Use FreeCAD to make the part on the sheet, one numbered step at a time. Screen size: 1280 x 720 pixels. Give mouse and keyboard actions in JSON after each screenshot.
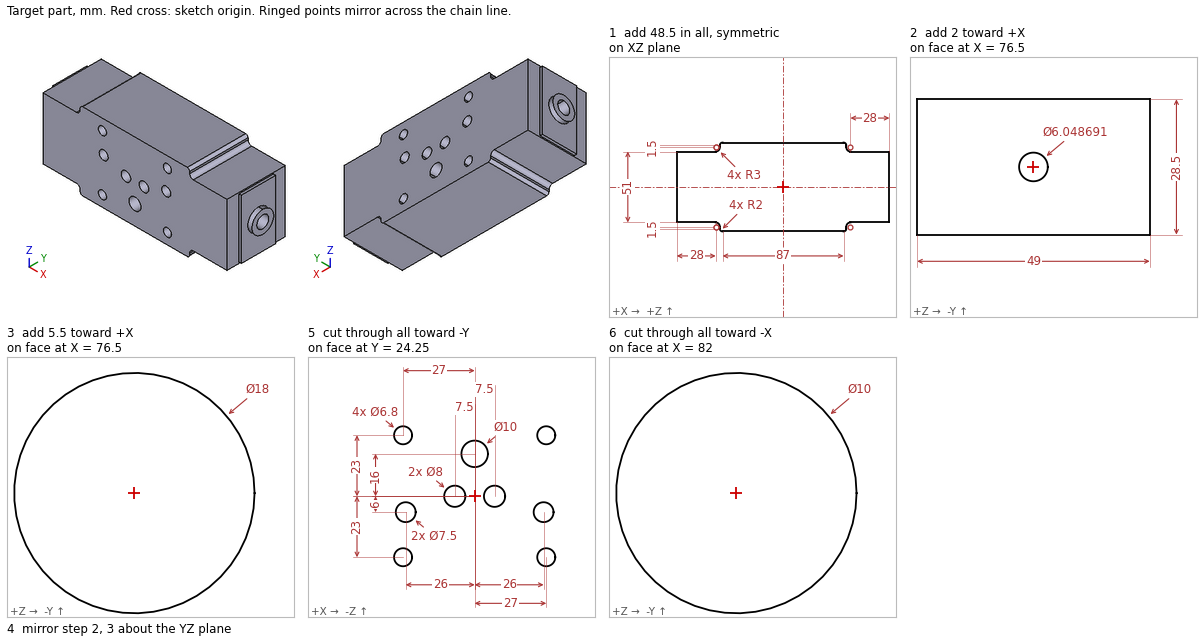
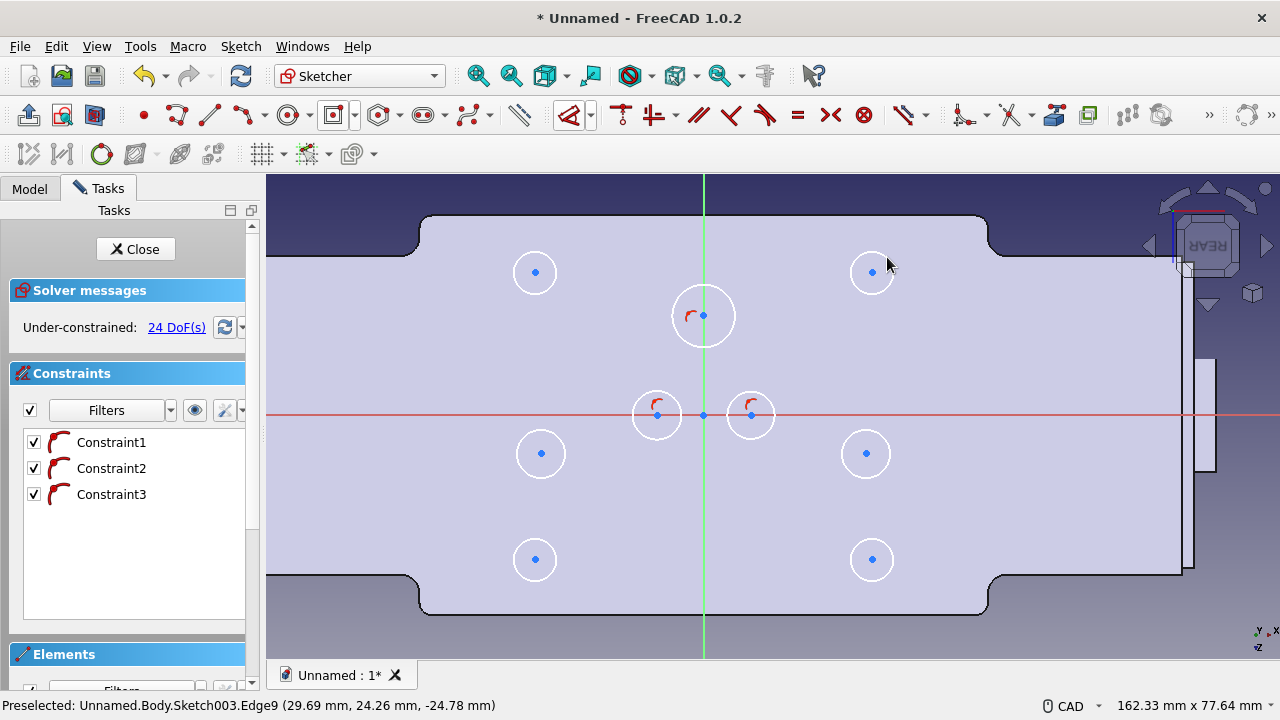
{"action": "left_click", "coordinate": [550, 258]}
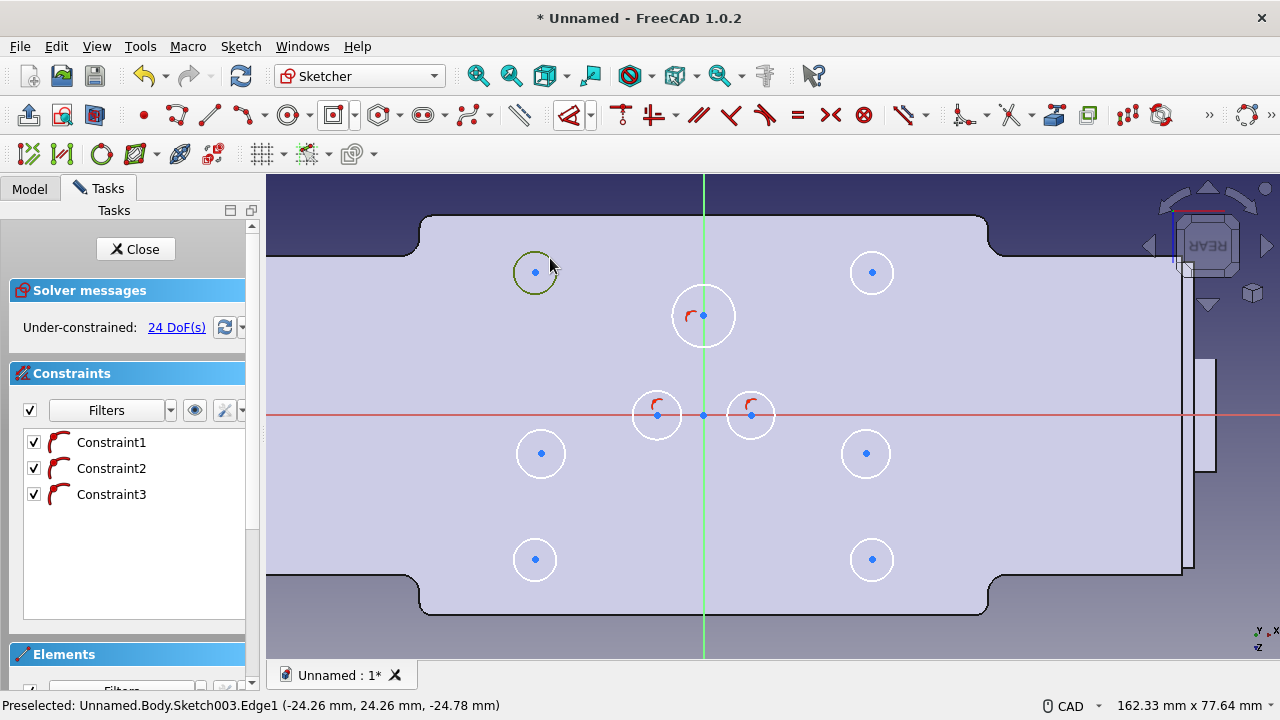
{"action": "left_click", "coordinate": [550, 545]}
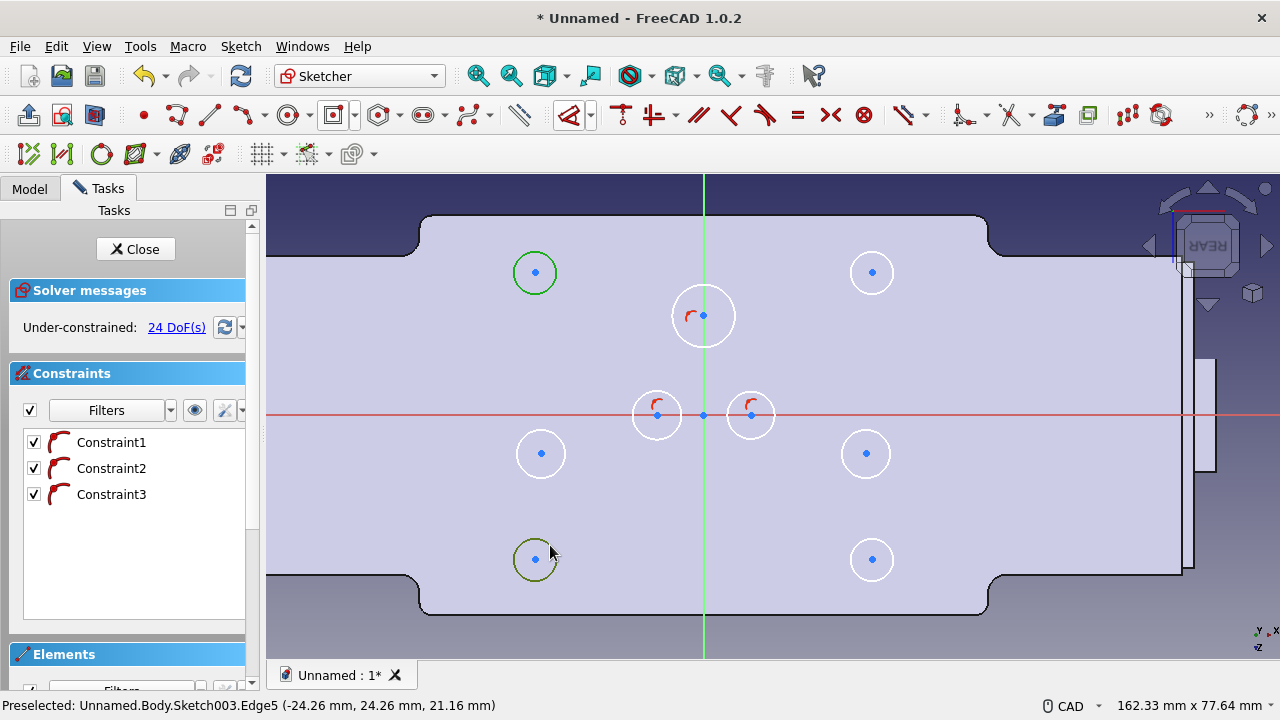
{"action": "left_click", "coordinate": [887, 545]}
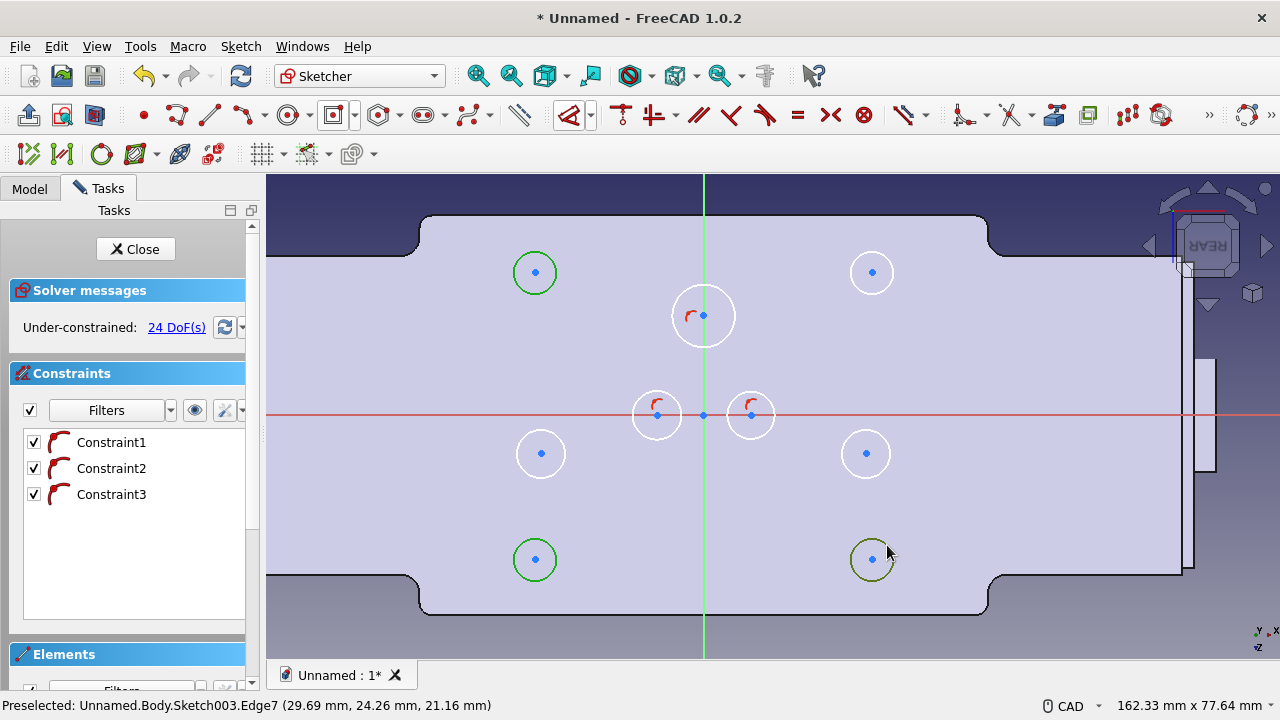
{"action": "left_click", "coordinate": [887, 258]}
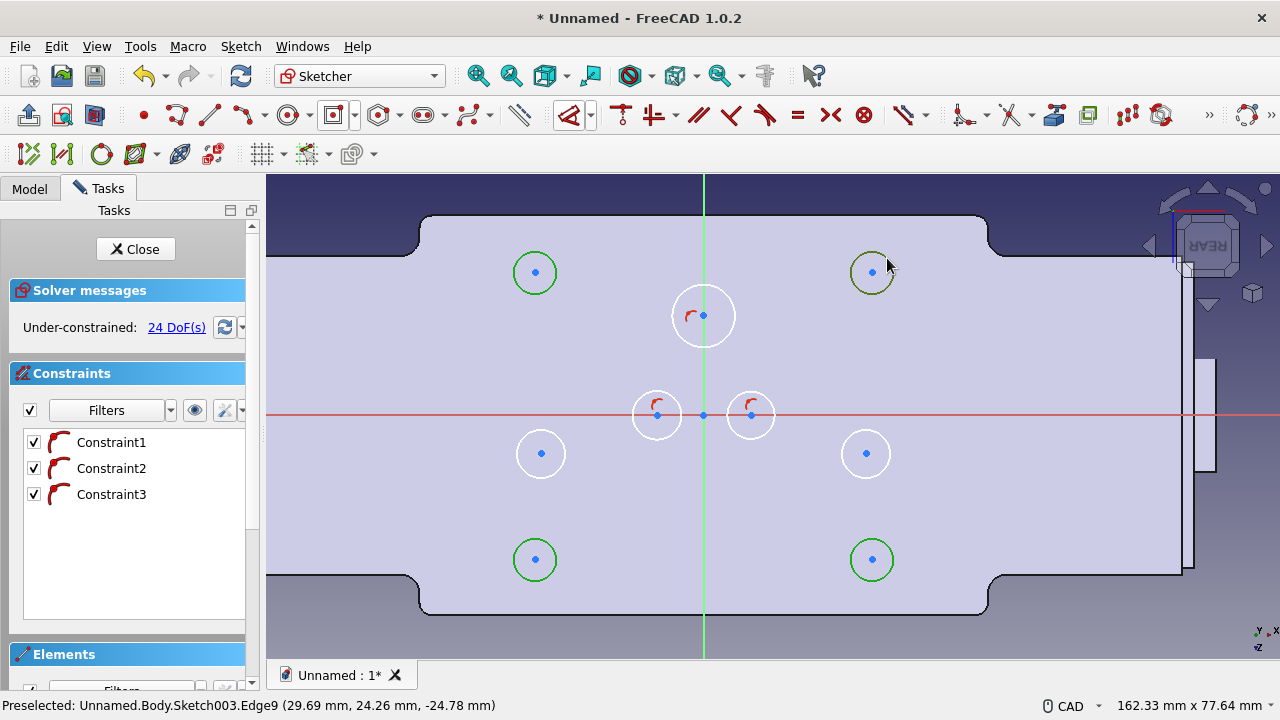
{"action": "left_click", "coordinate": [798, 116]}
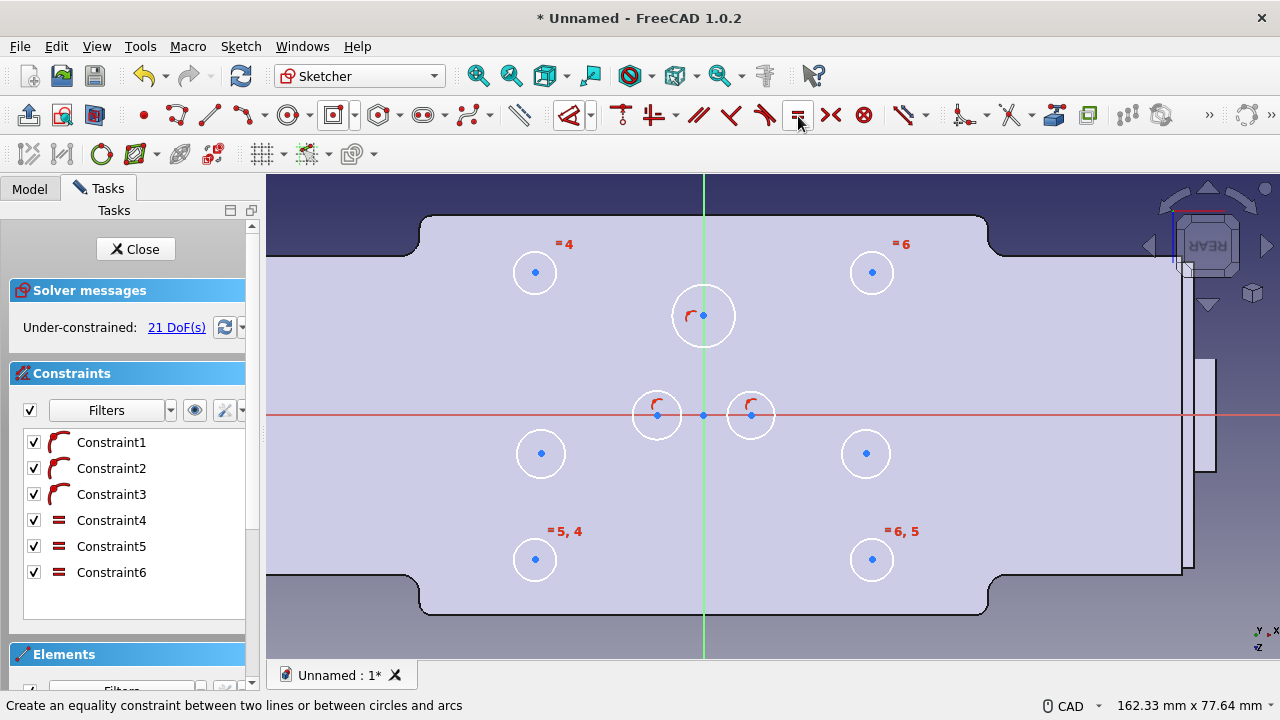
{"action": "left_click", "coordinate": [674, 398]}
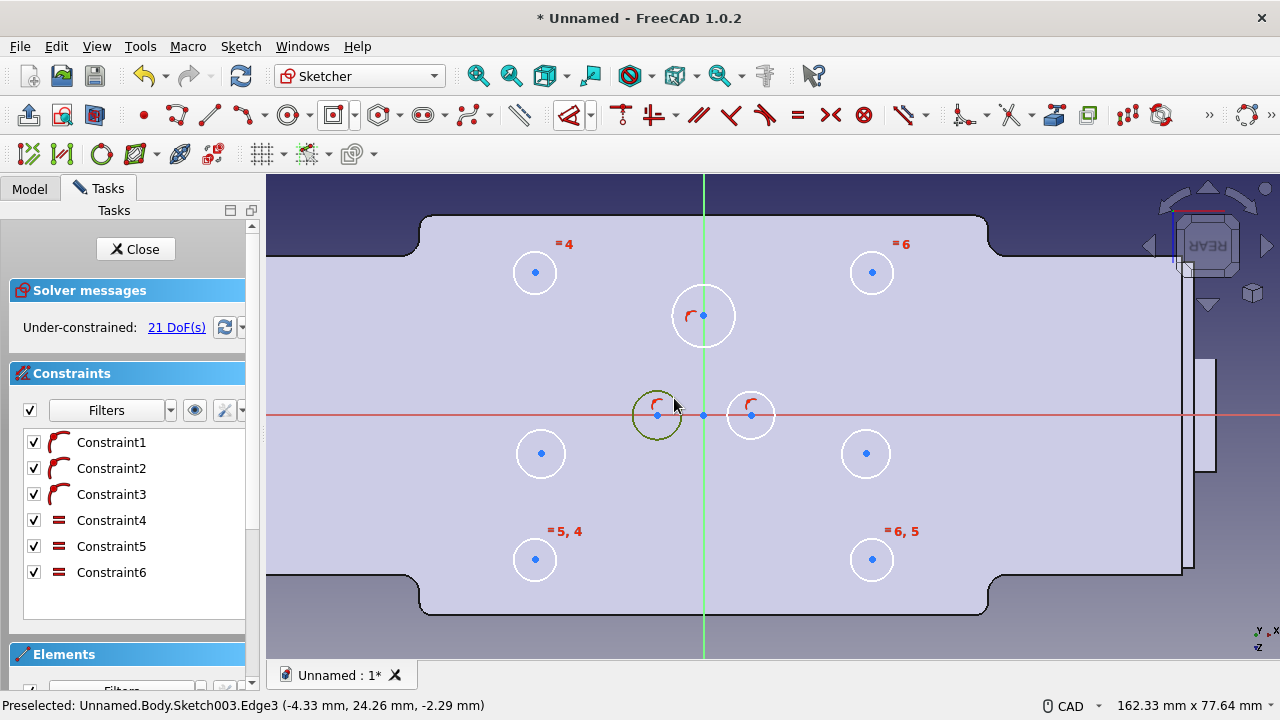
{"action": "left_click", "coordinate": [768, 399]}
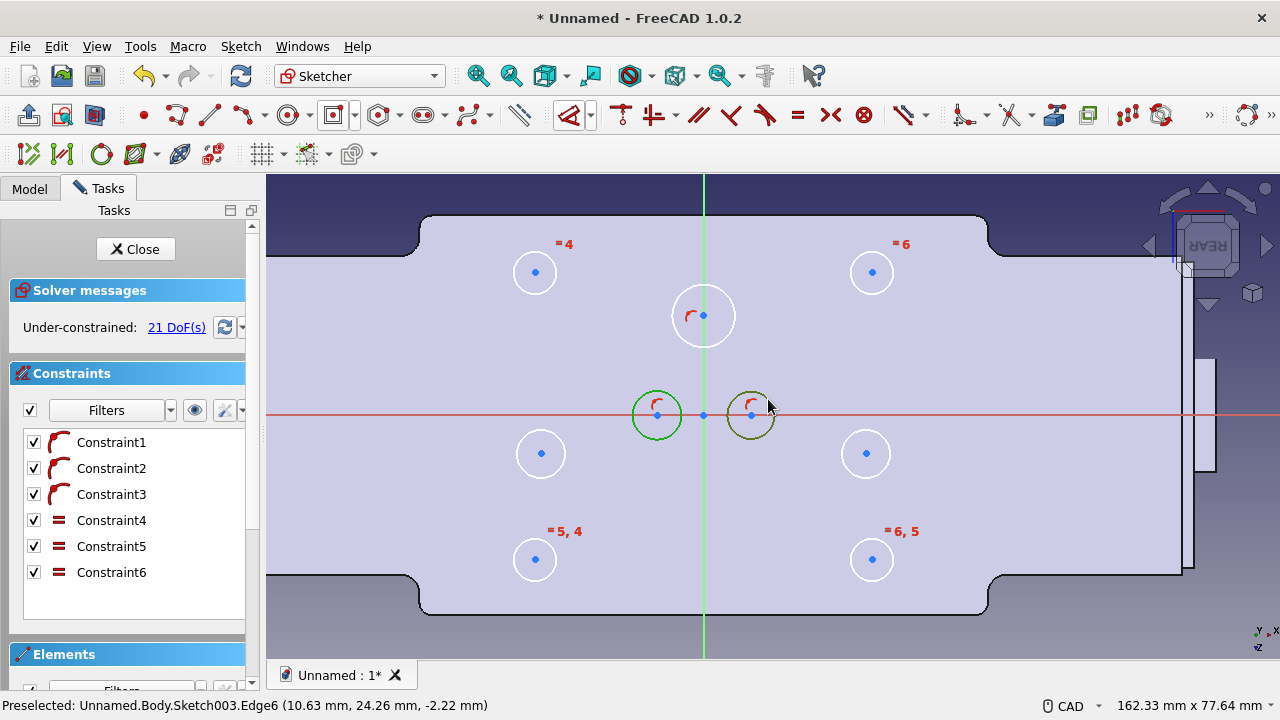
{"action": "left_click", "coordinate": [798, 116]}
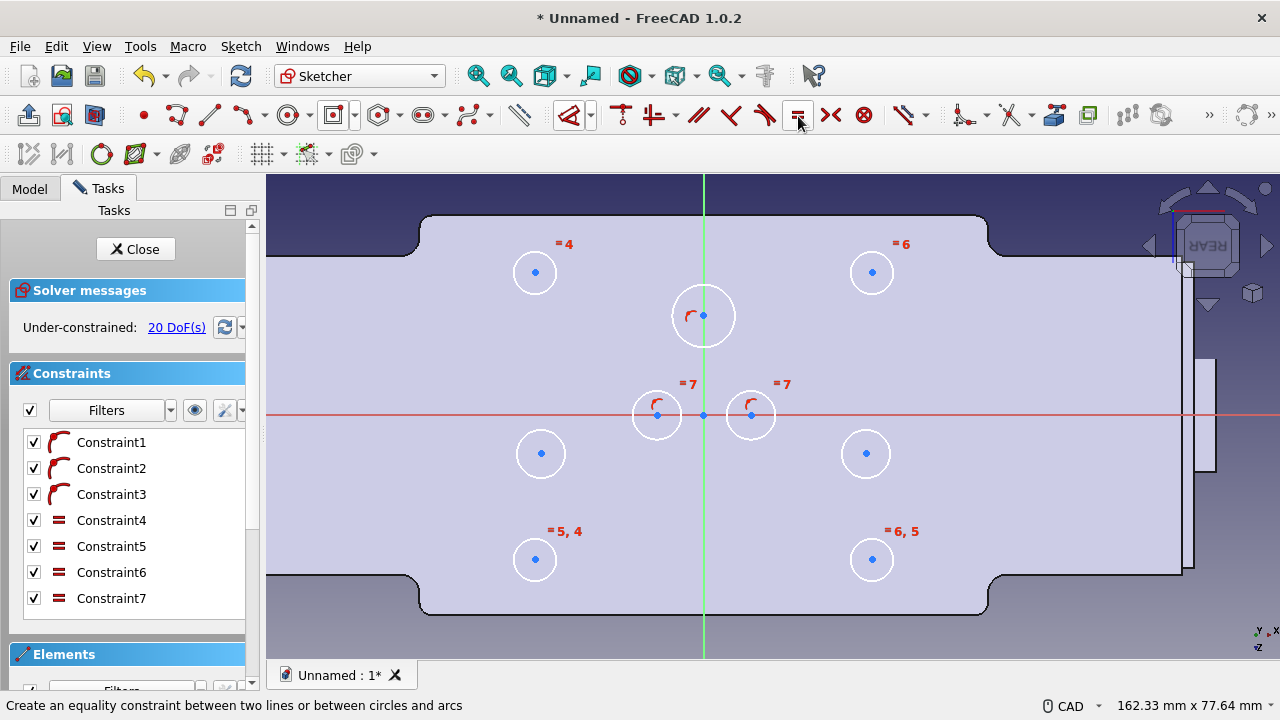
{"action": "left_click", "coordinate": [558, 437]}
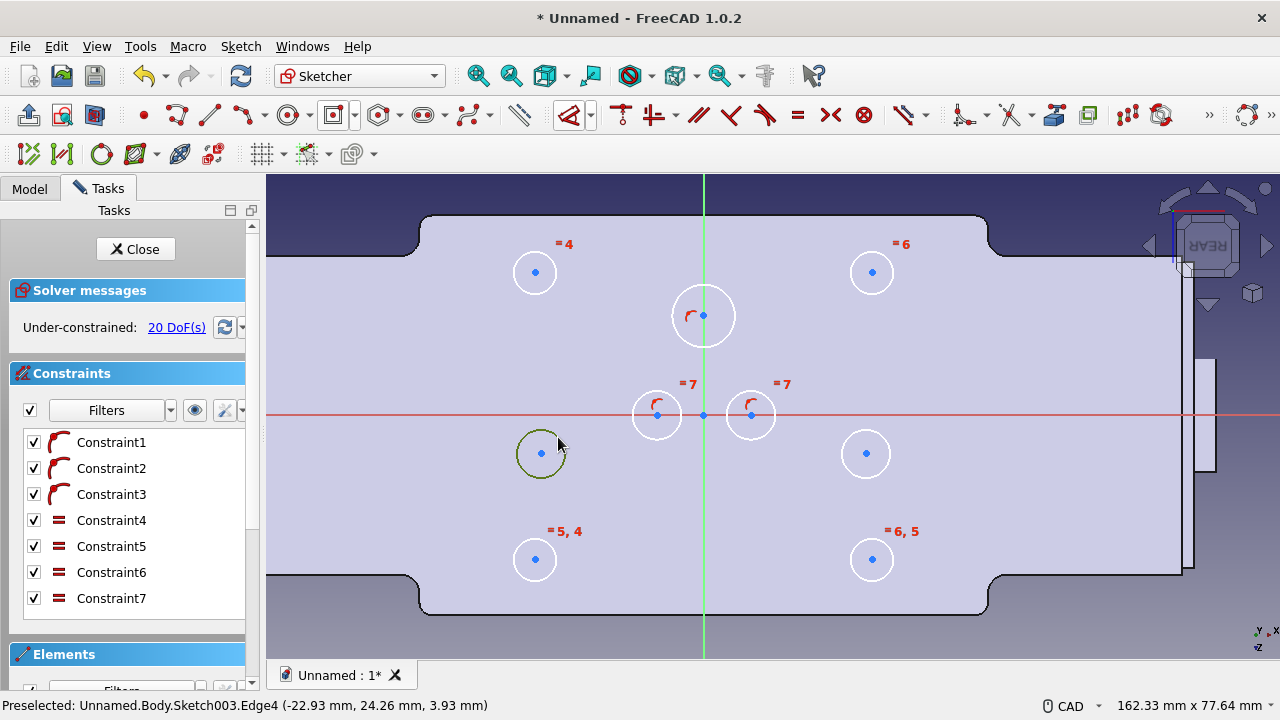
{"action": "left_click", "coordinate": [883, 437]}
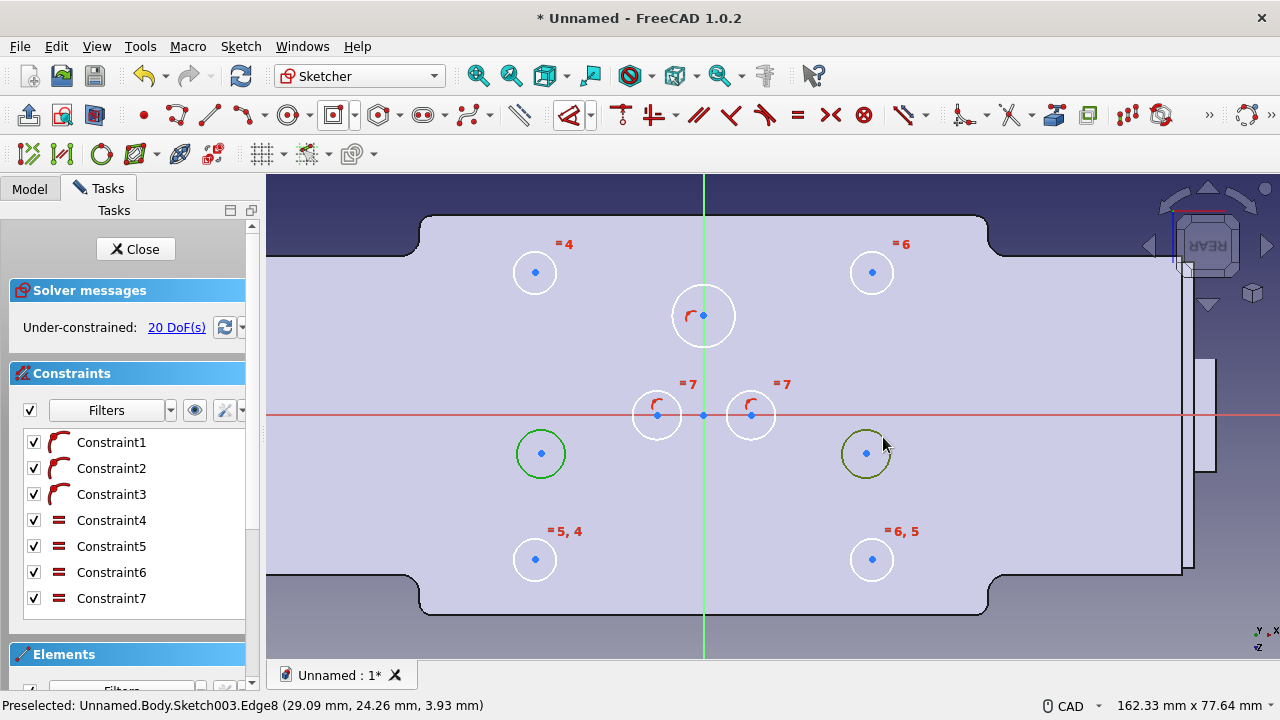
{"action": "left_click", "coordinate": [798, 116]}